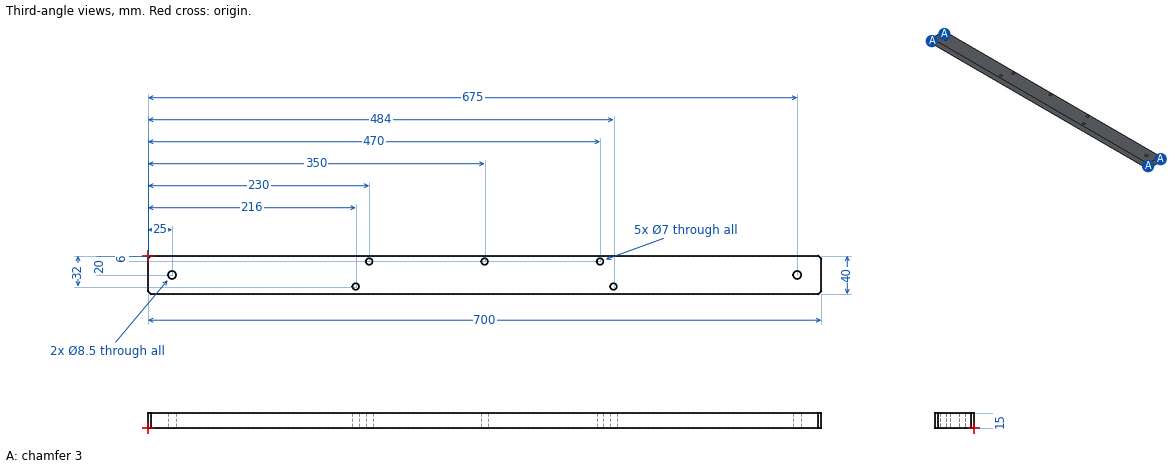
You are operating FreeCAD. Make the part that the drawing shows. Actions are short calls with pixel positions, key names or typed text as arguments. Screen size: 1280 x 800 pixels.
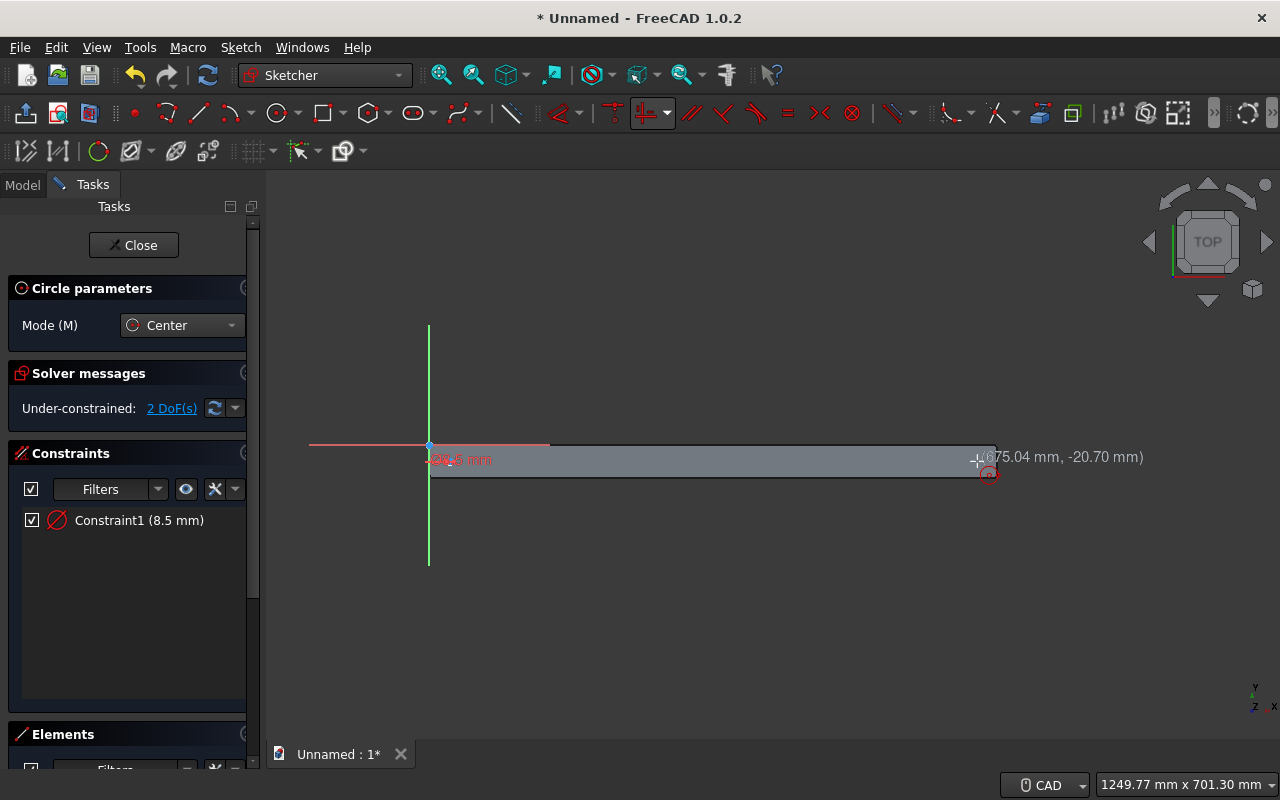
click(977, 461)
move(979, 464)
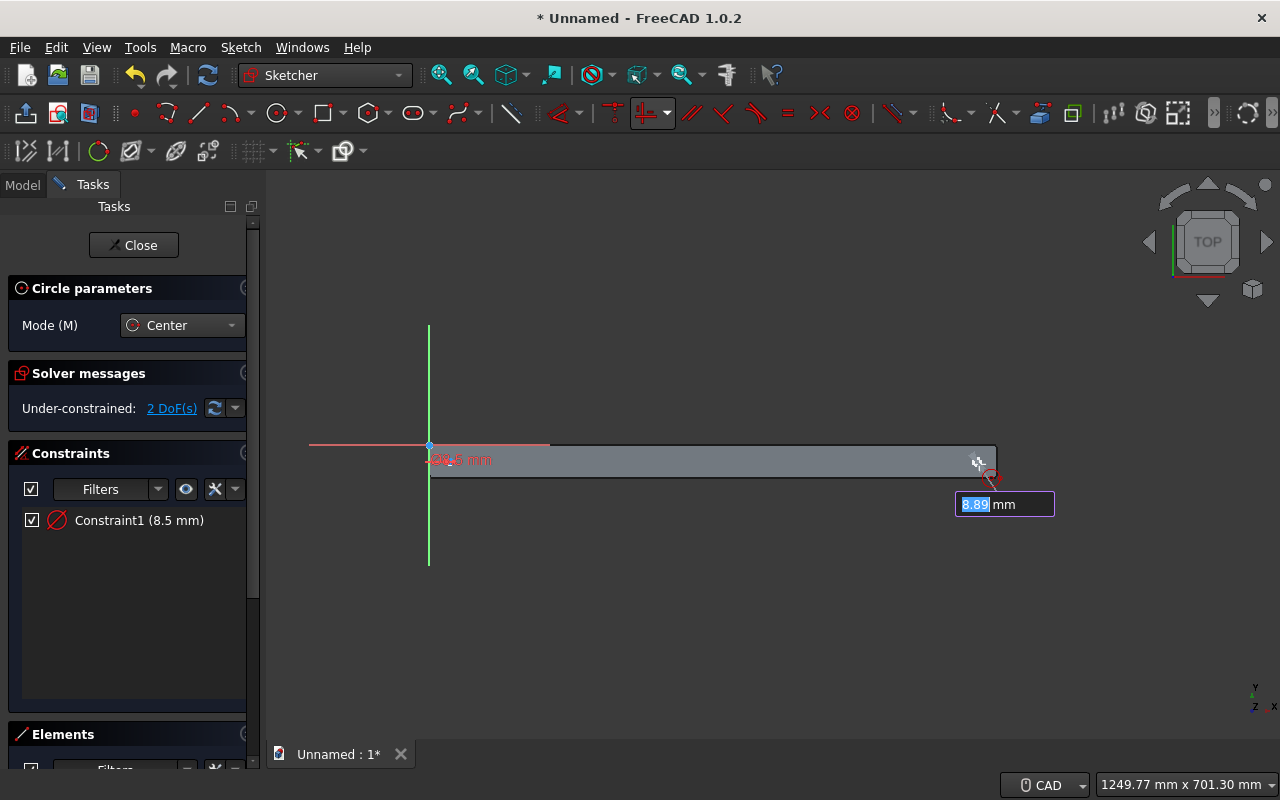
text(8.5)
key(Return)
key(Escape)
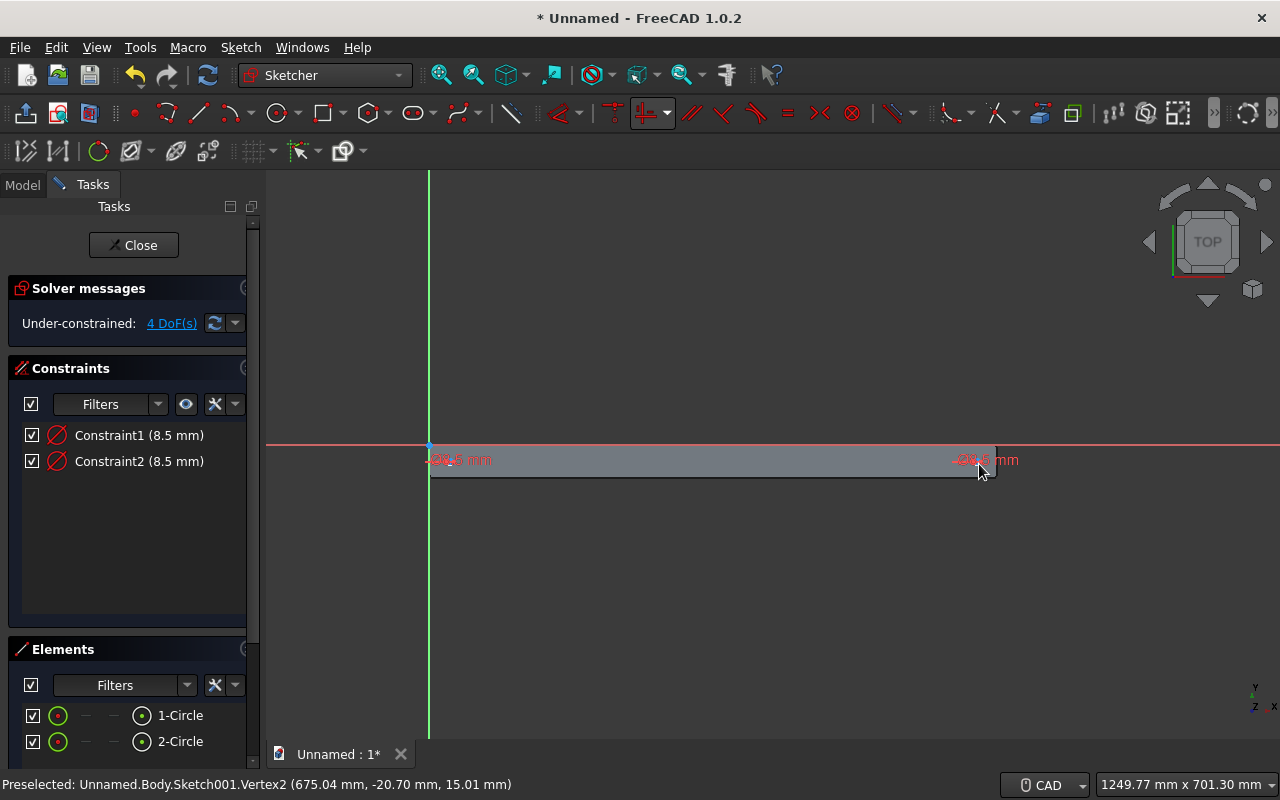
click(450, 462)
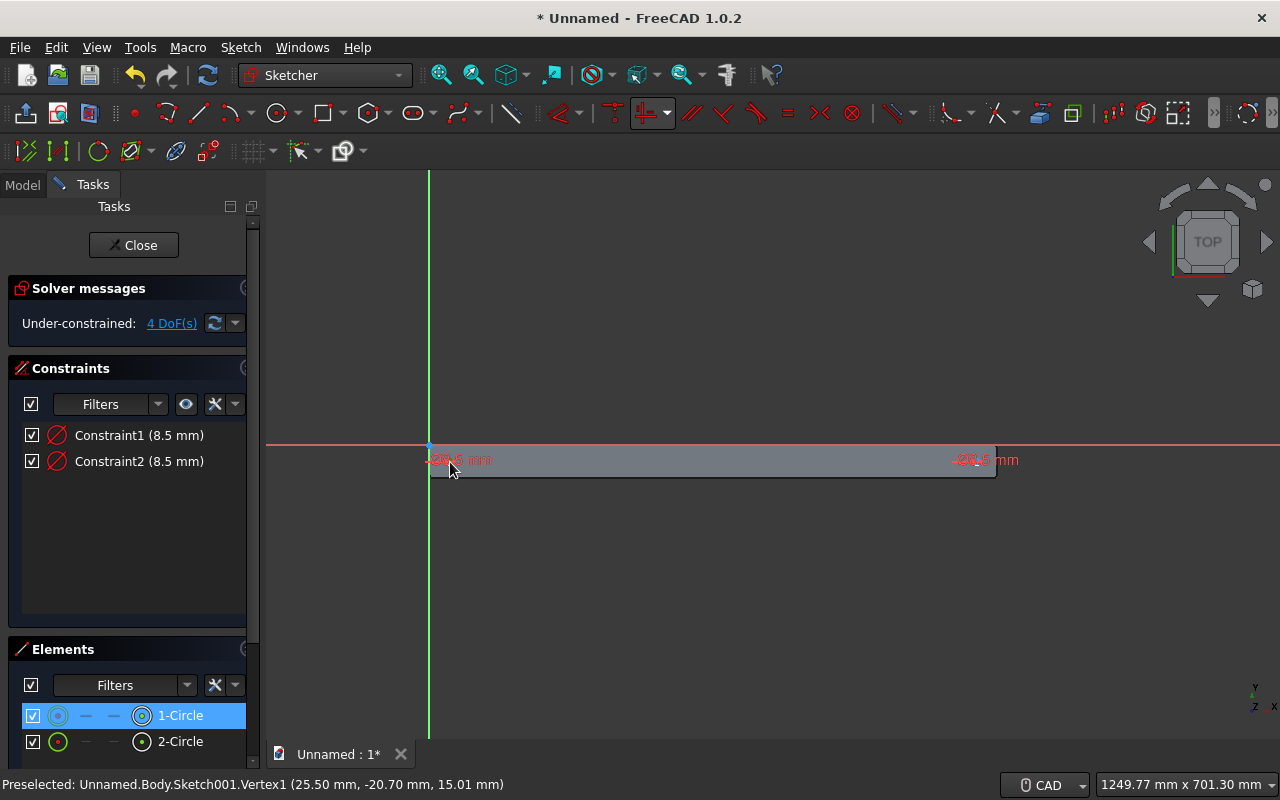
click(977, 462)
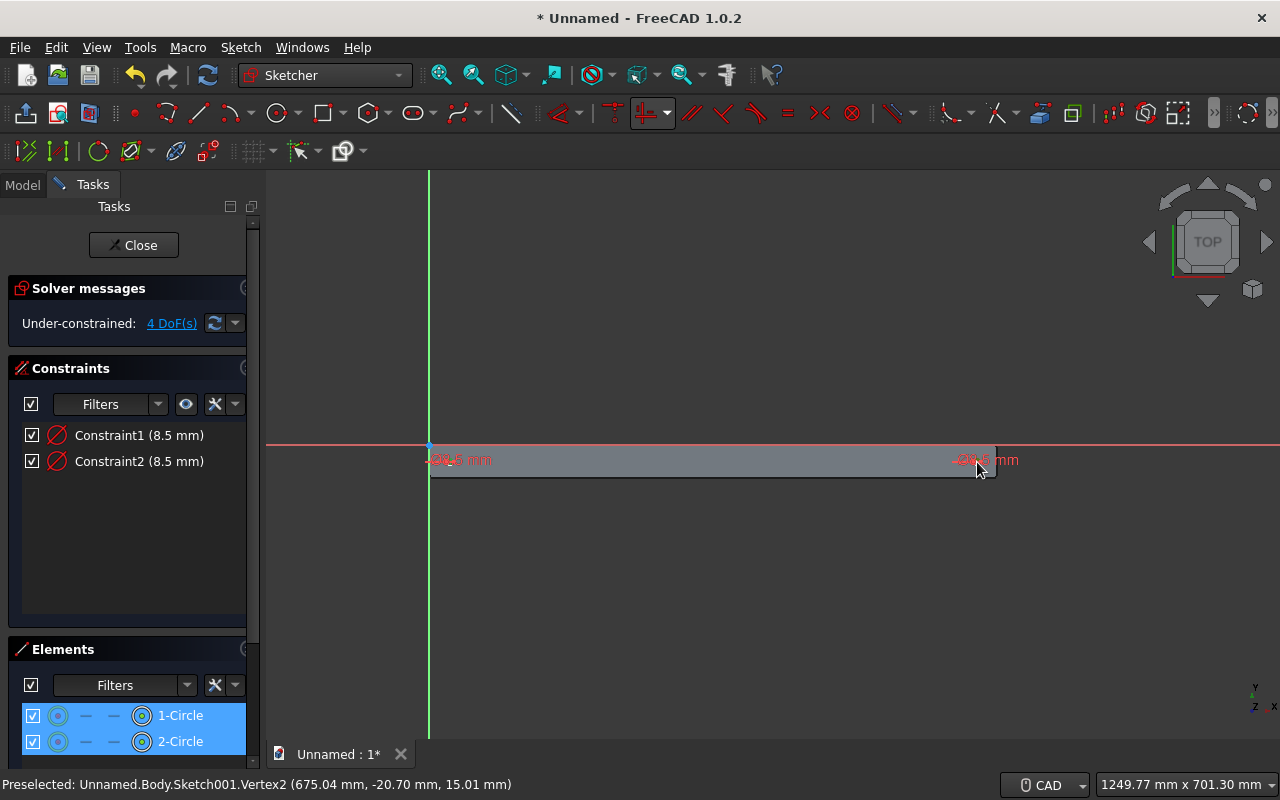
key(h)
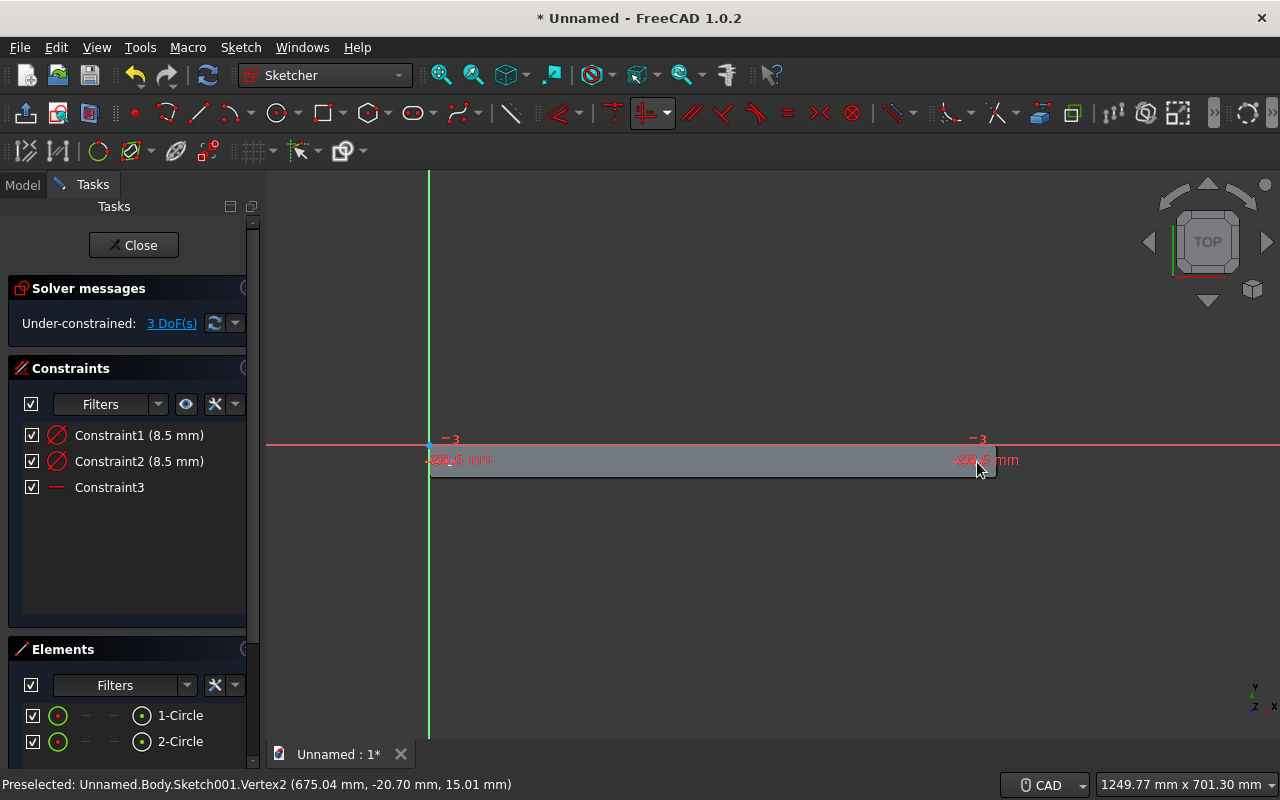
click(558, 114)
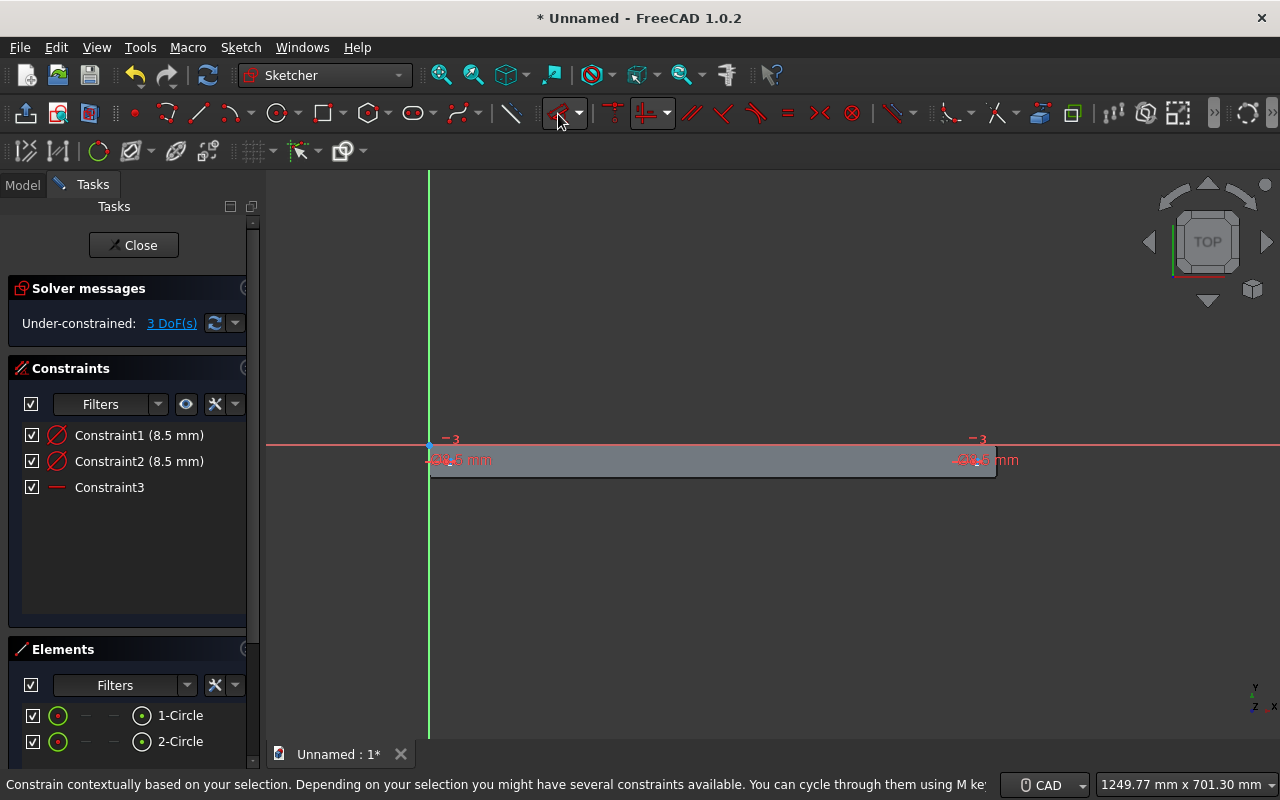
scroll(450, 462, up, 4)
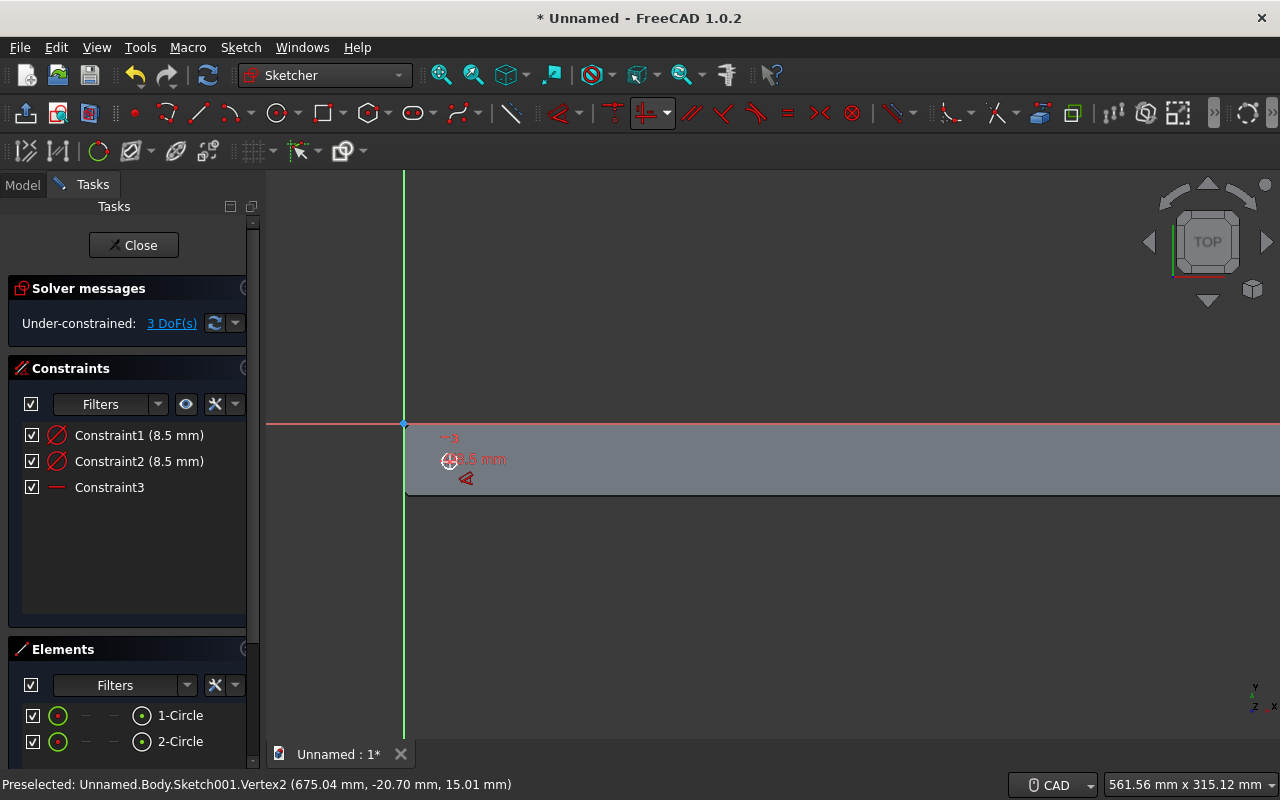
click(450, 461)
click(427, 390)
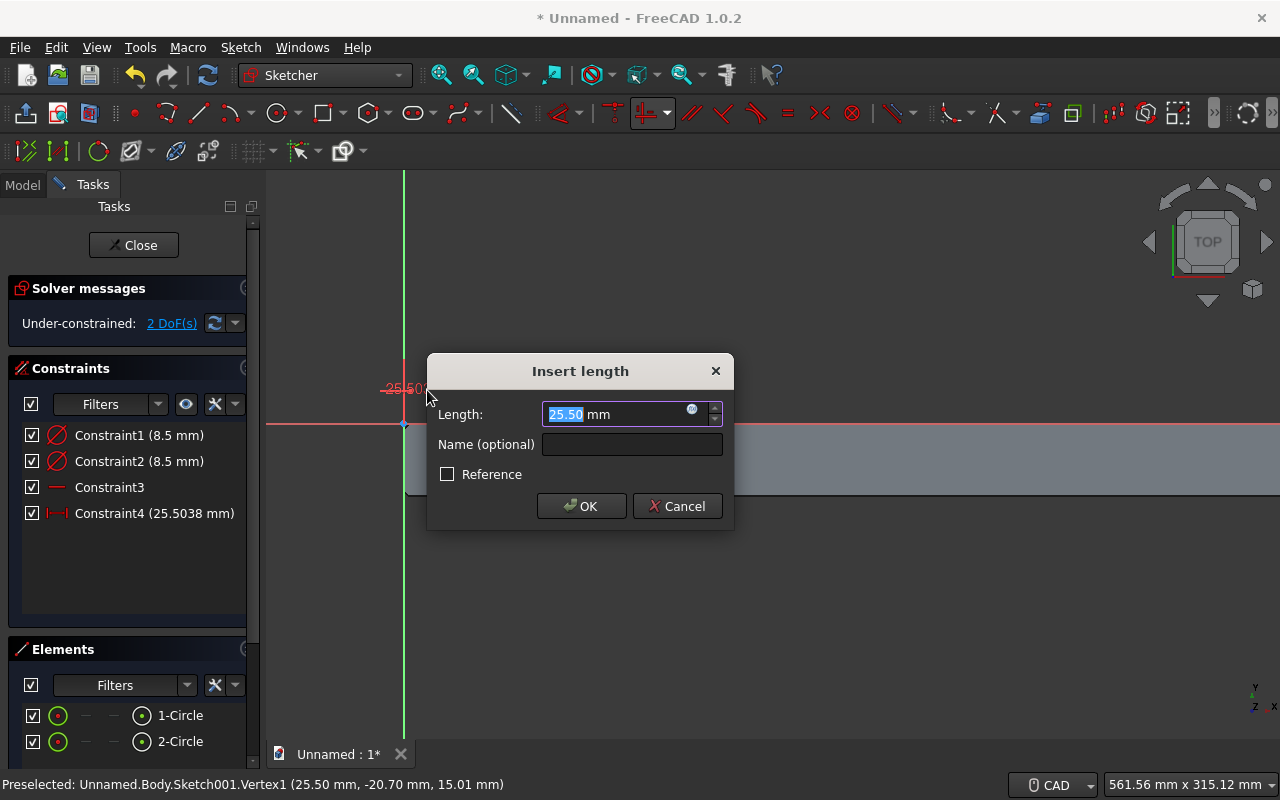
text(25)
key(Return)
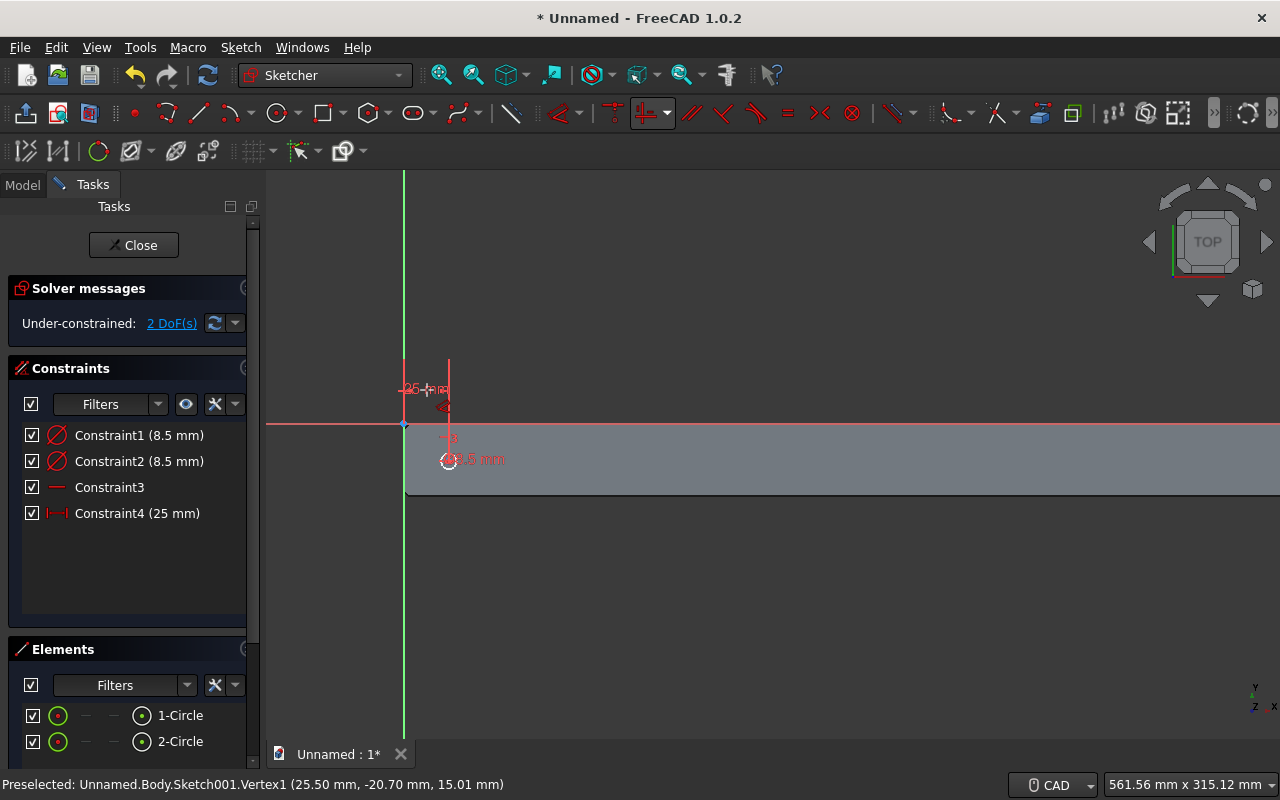
click(449, 461)
click(370, 443)